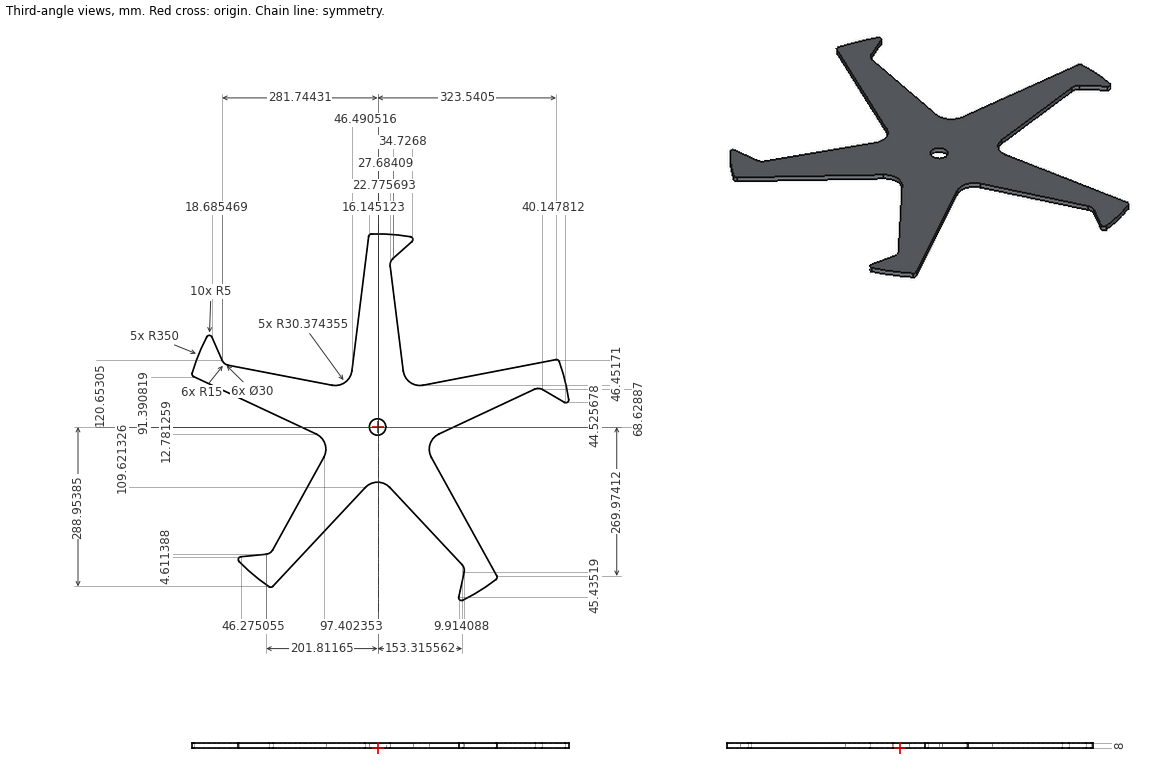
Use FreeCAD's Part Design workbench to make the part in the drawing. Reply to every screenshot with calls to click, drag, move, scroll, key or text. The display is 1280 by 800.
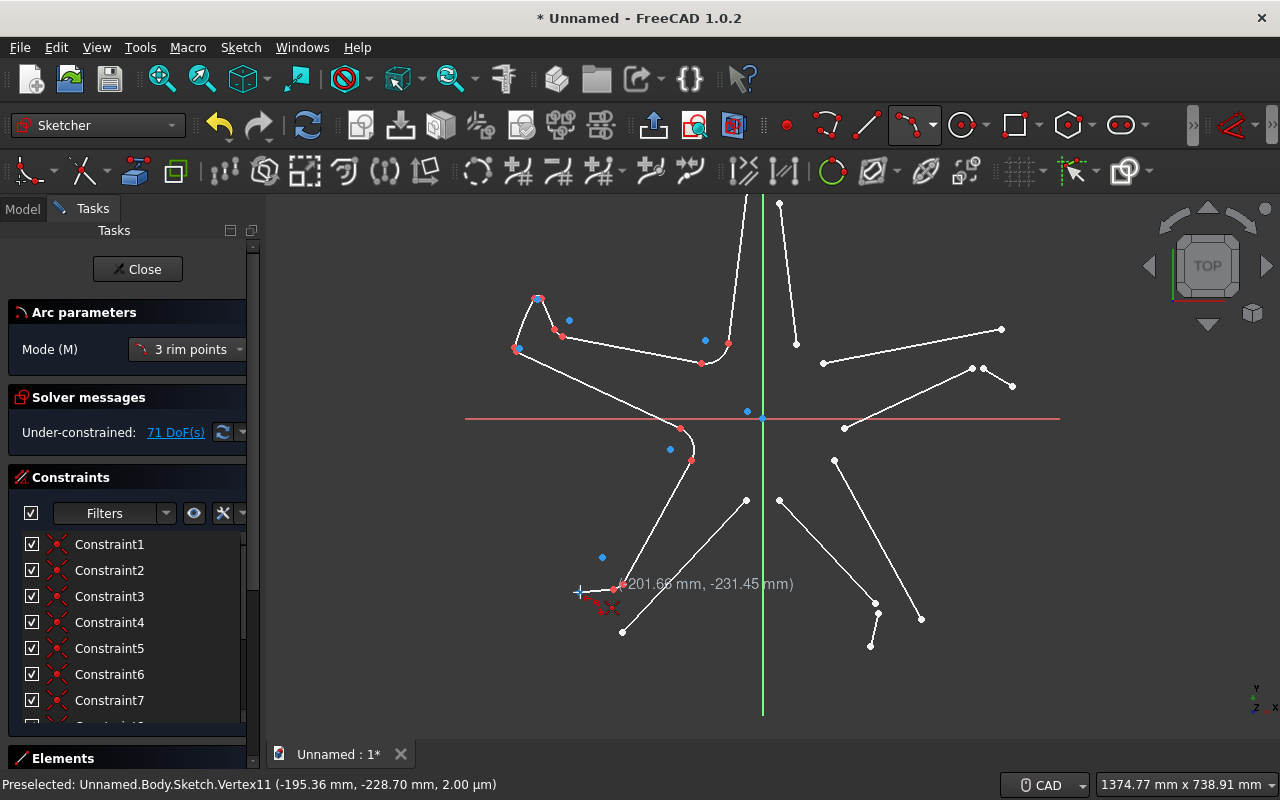
click(579, 593)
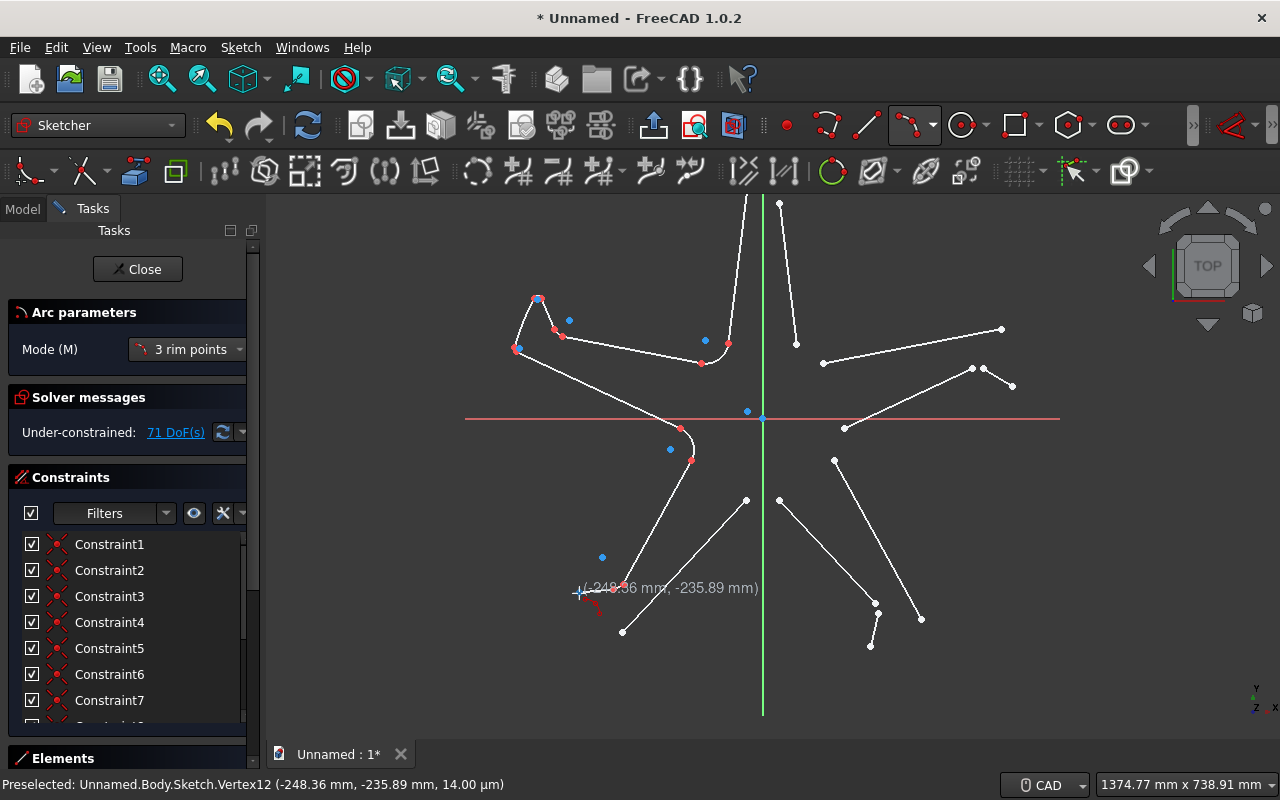
scroll(577, 598, up, 5)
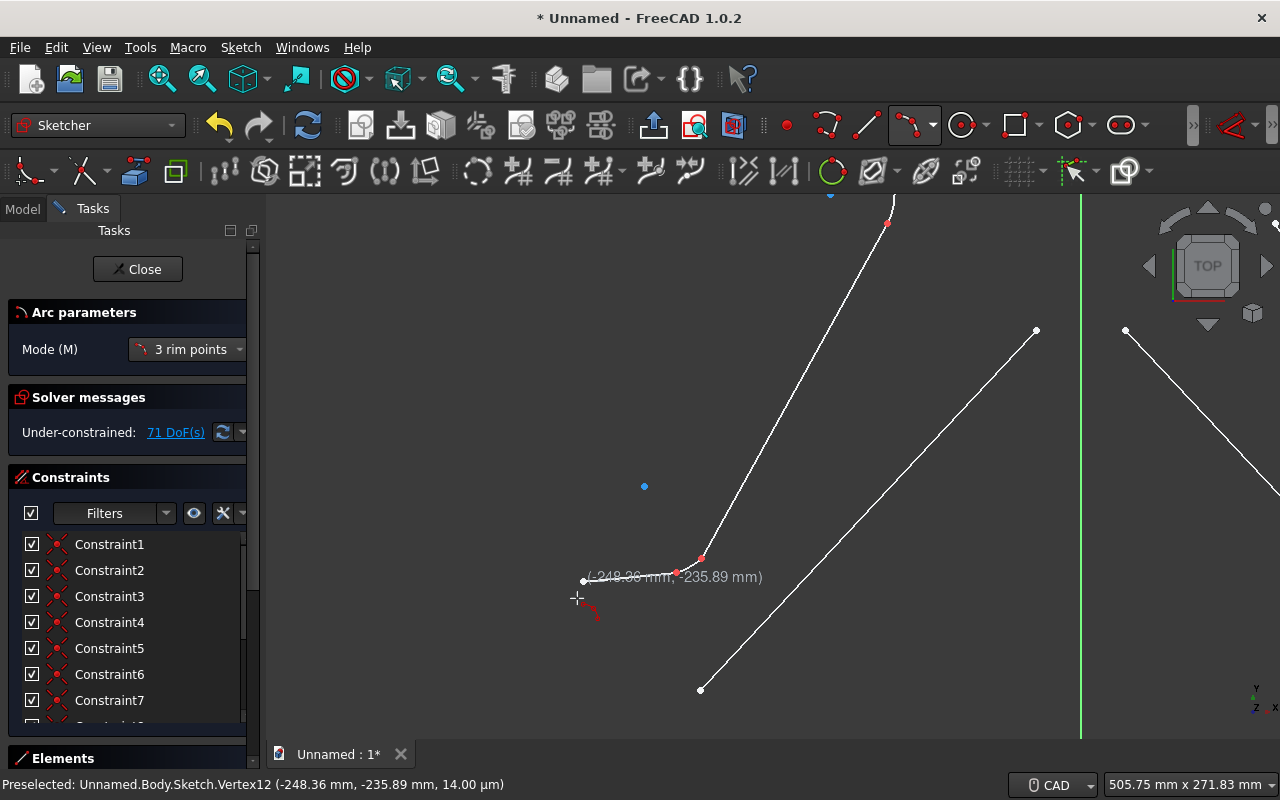
click(577, 598)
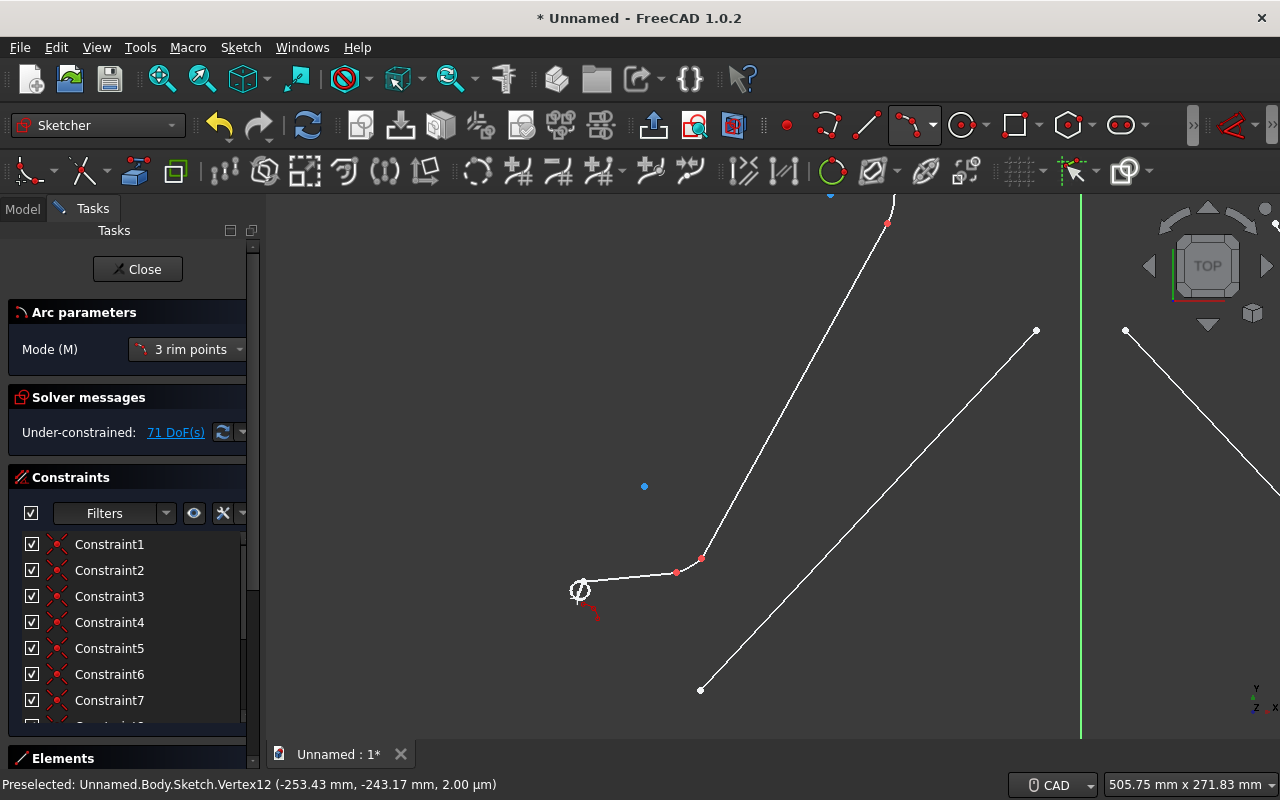
scroll(575, 587, up, 6)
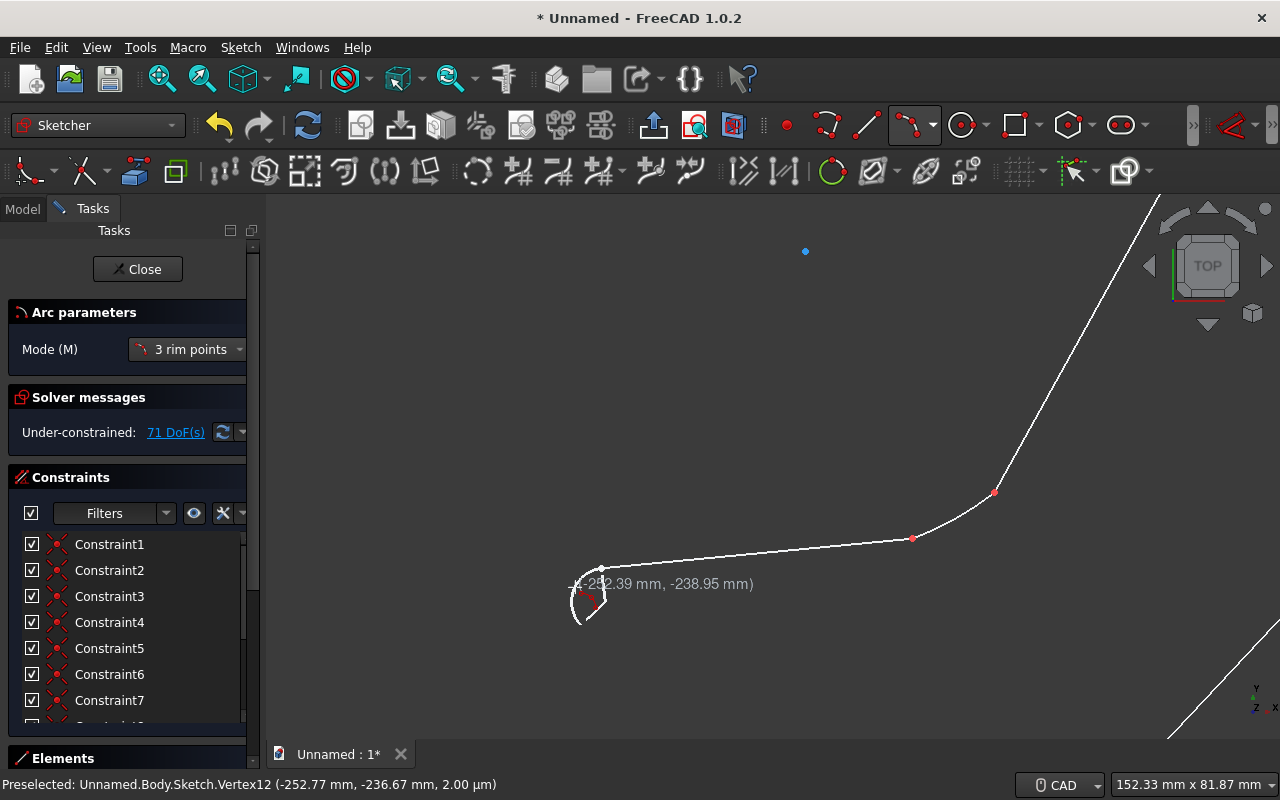
click(575, 586)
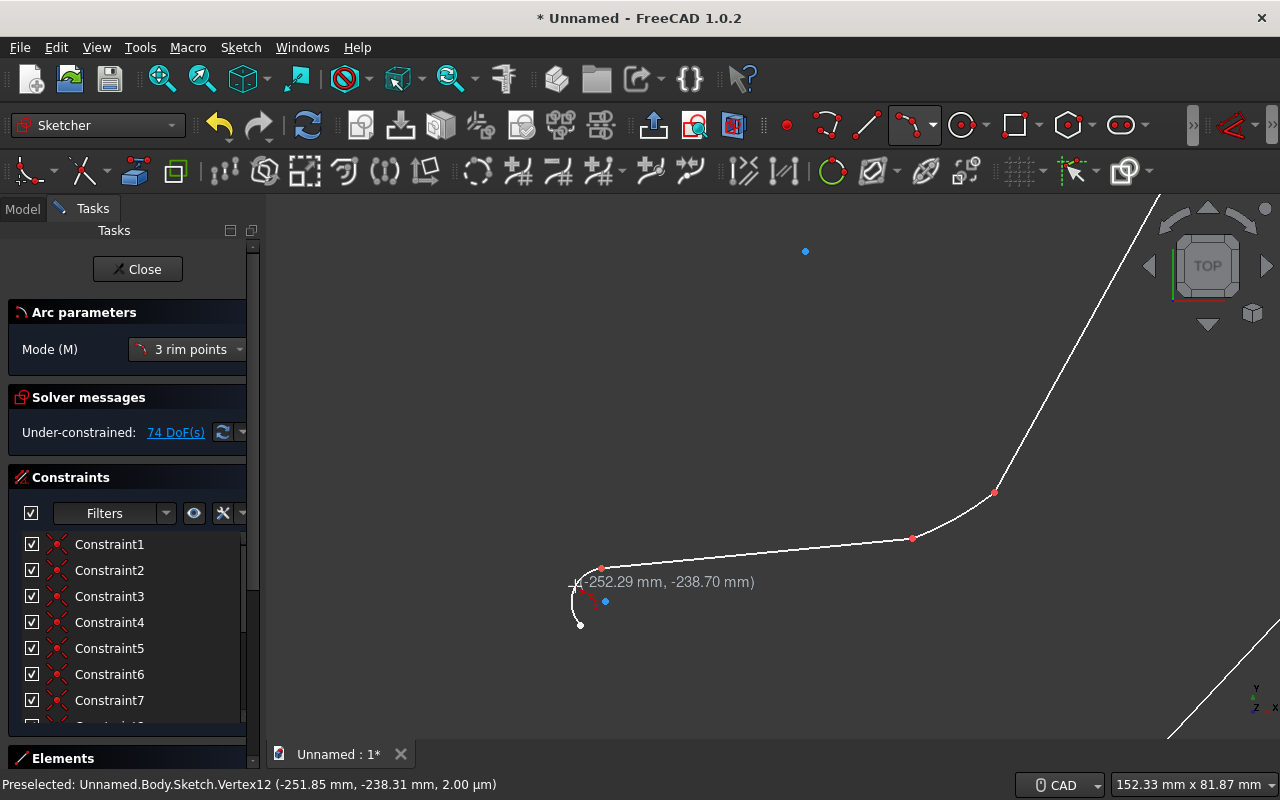
click(581, 625)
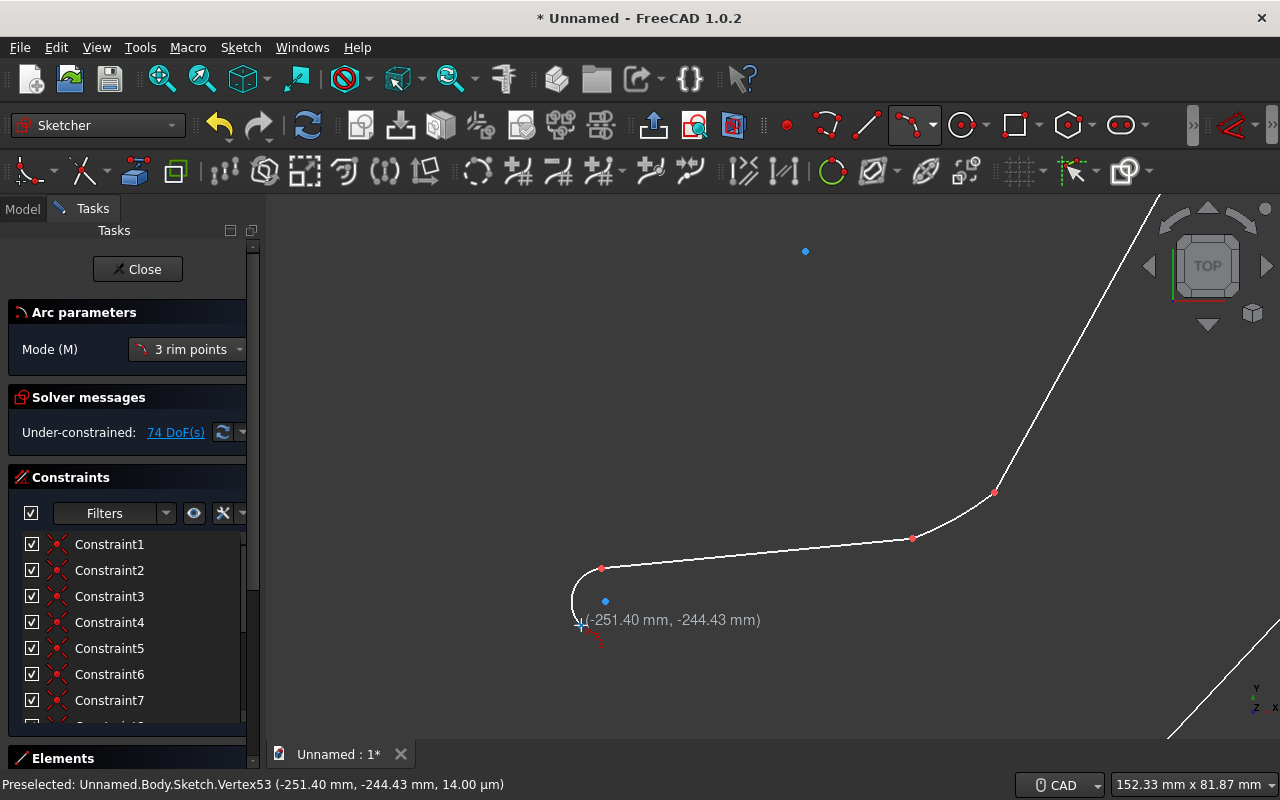
scroll(577, 594, down, 13)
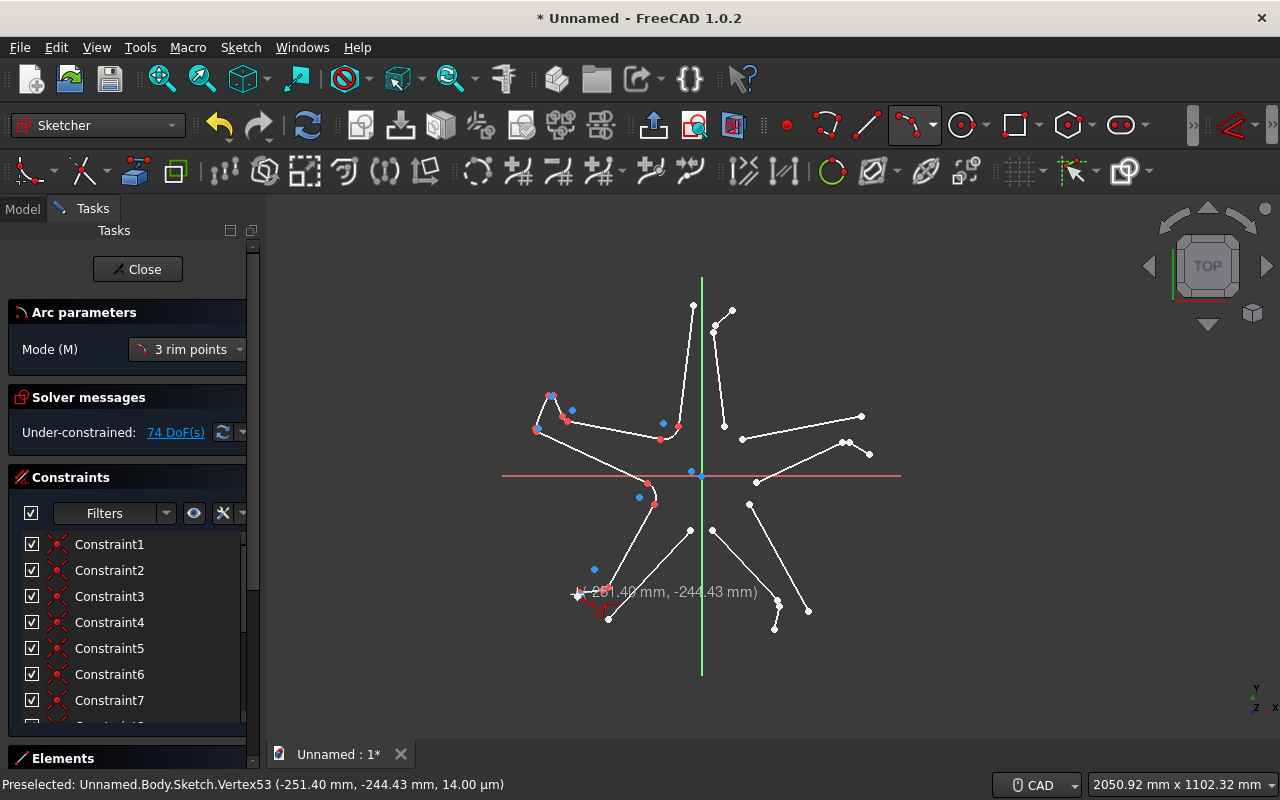
scroll(605, 619, up, 8)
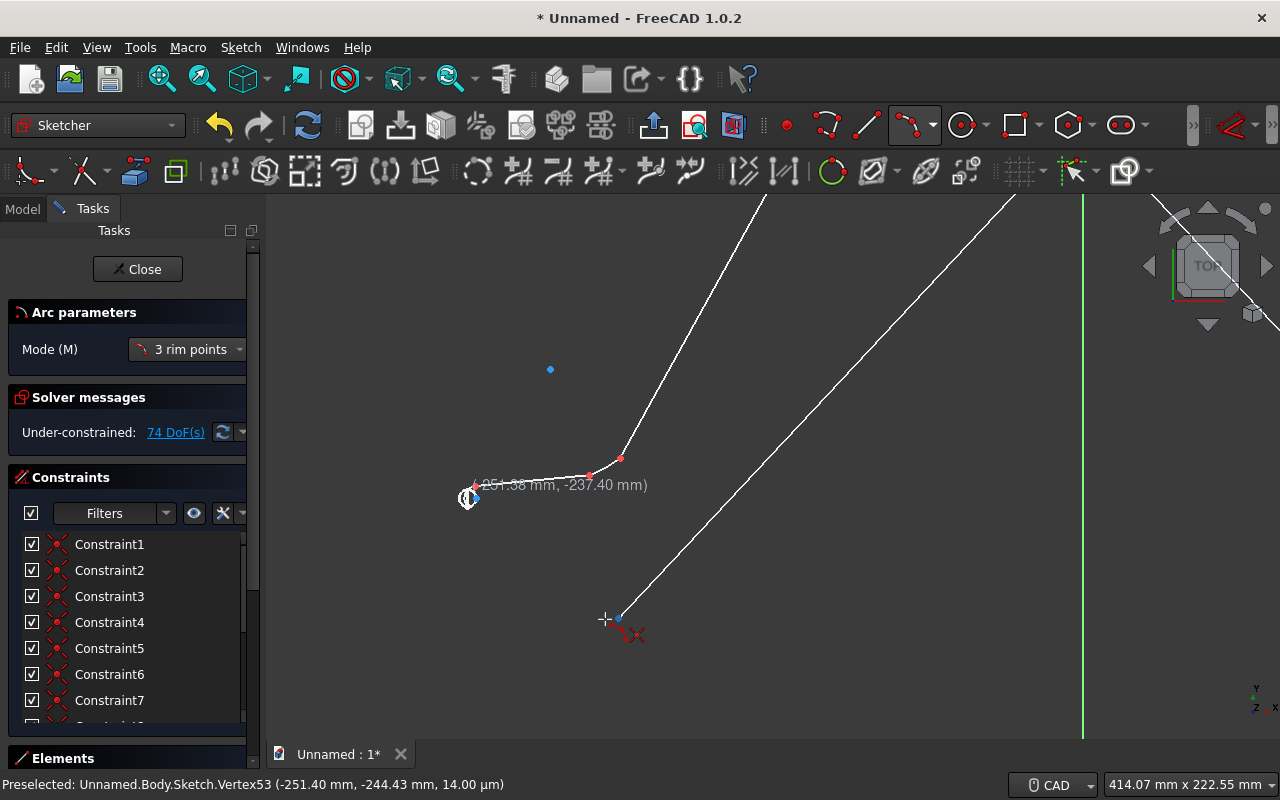
click(602, 618)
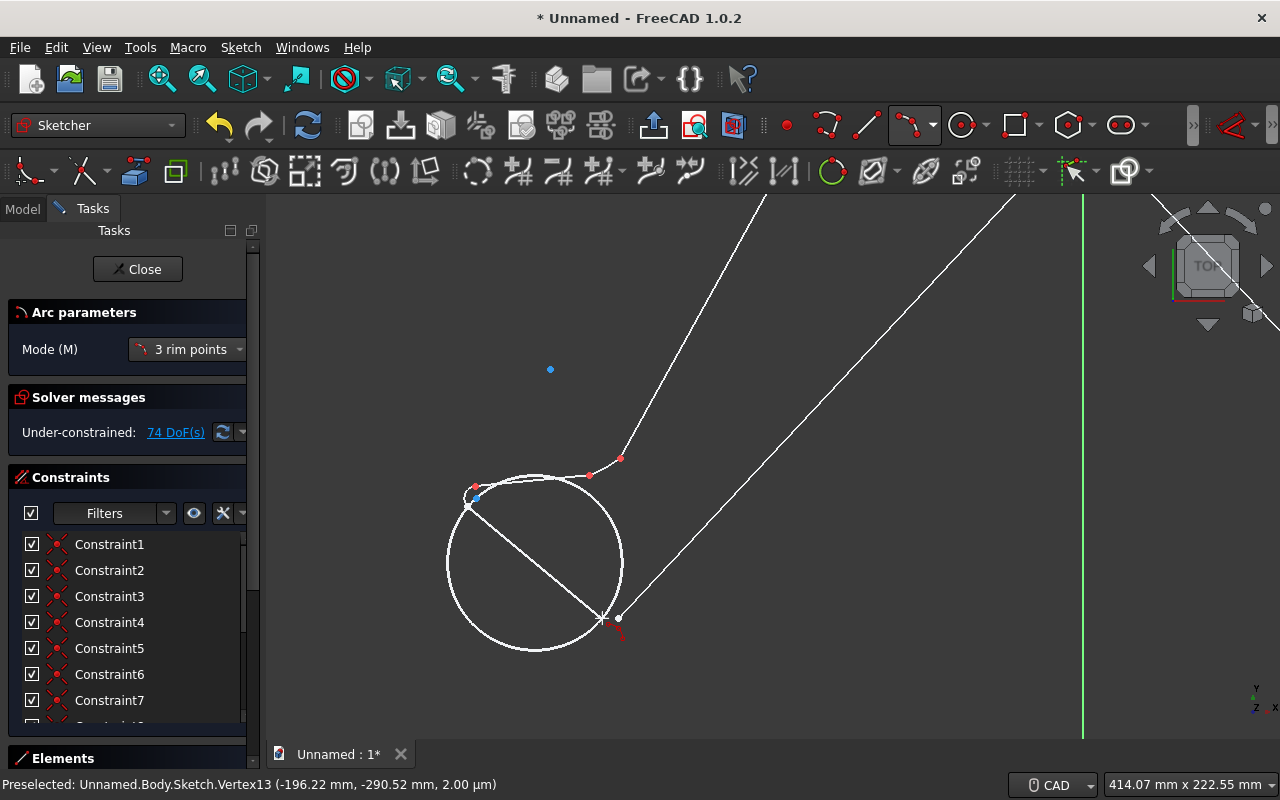
scroll(533, 565, up, 7)